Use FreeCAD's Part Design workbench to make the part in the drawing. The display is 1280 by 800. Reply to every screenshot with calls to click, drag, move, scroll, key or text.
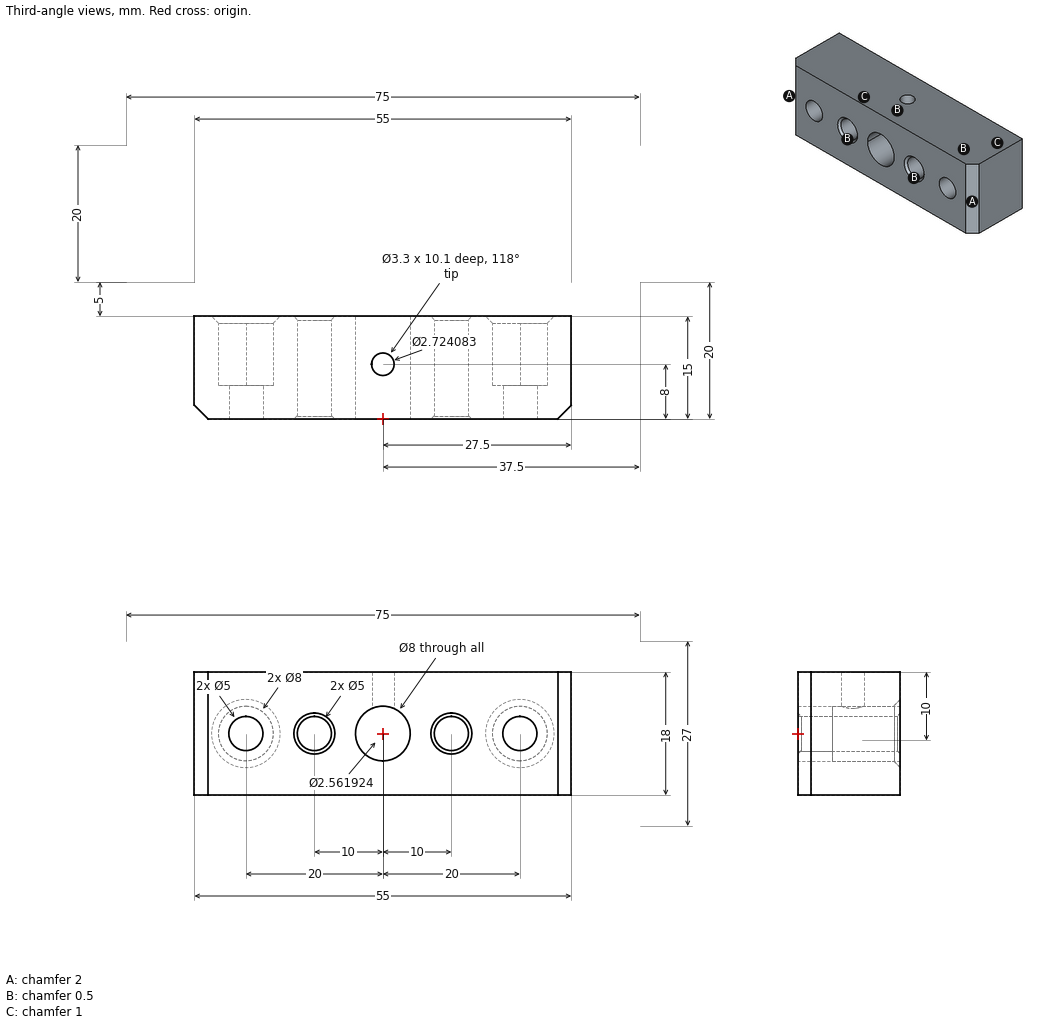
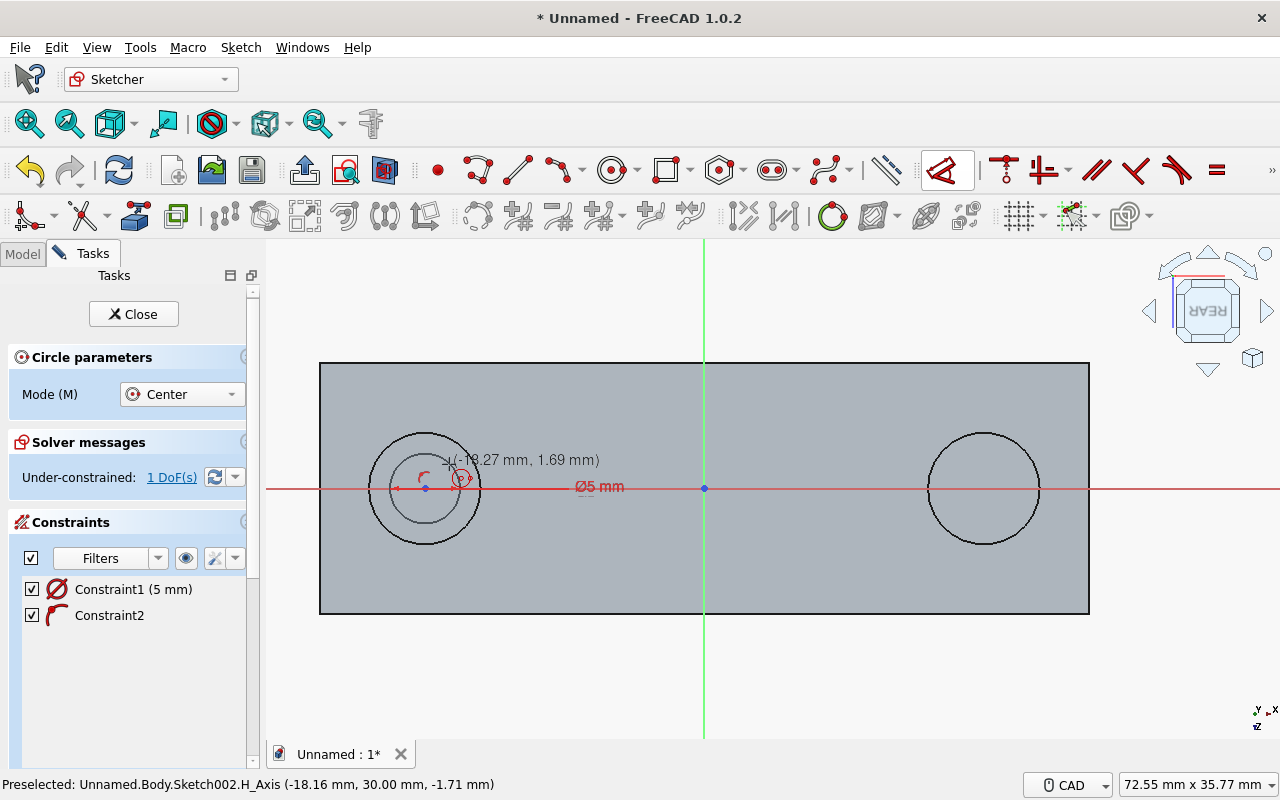
click(984, 489)
move(1009, 464)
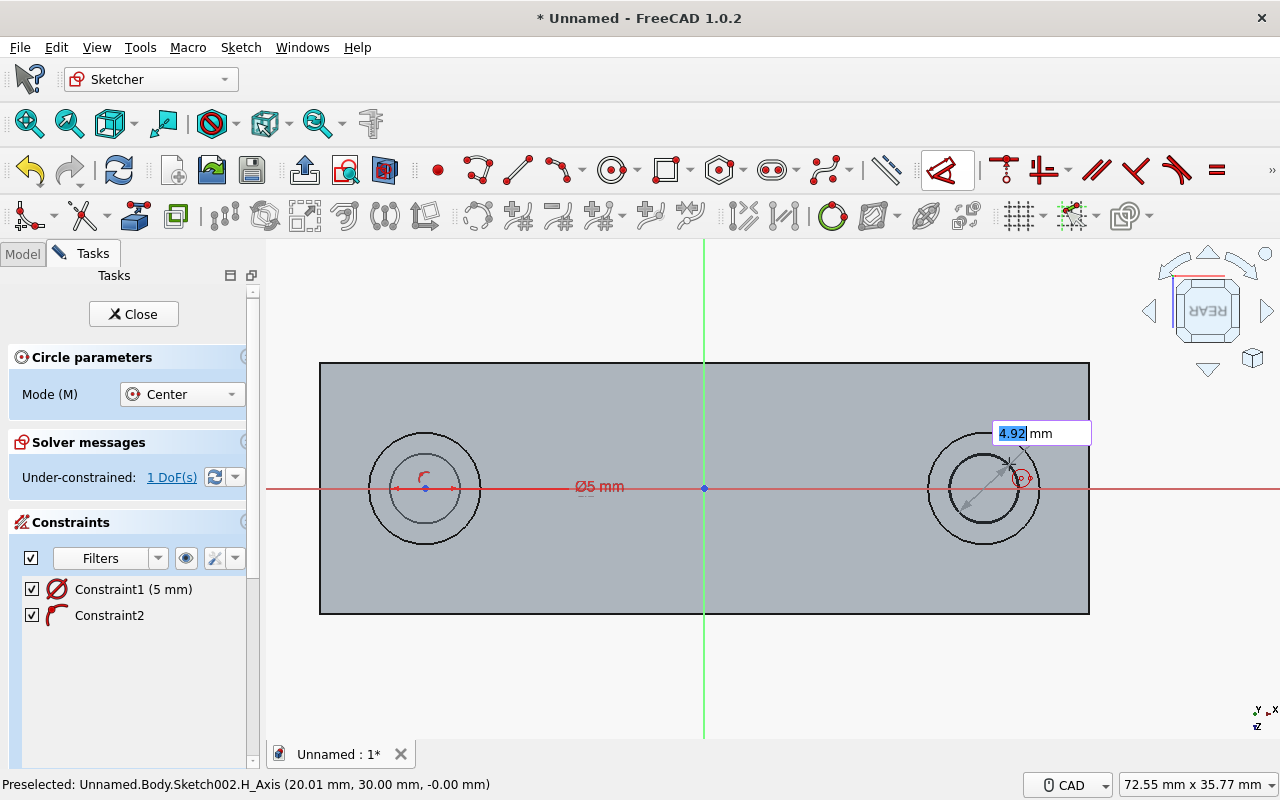
text(5)
key(Return)
key(Escape)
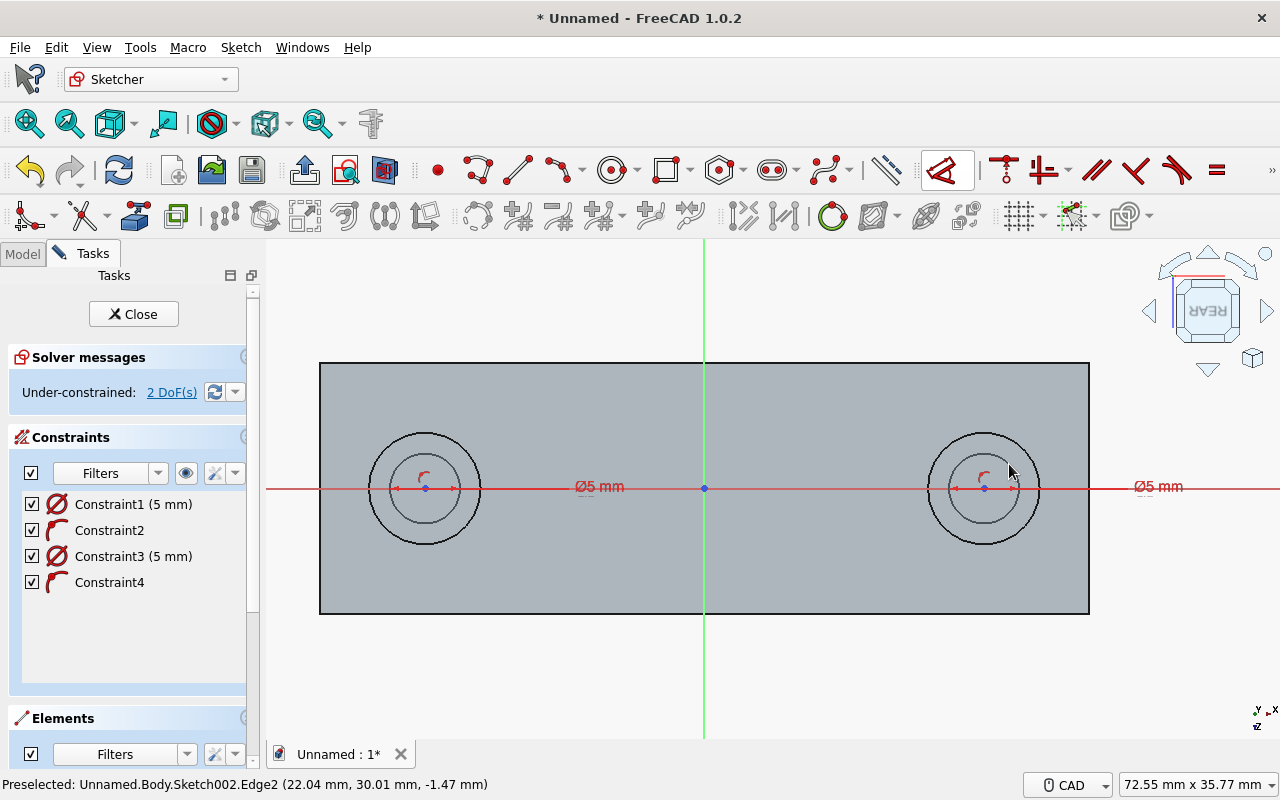
click(425, 489)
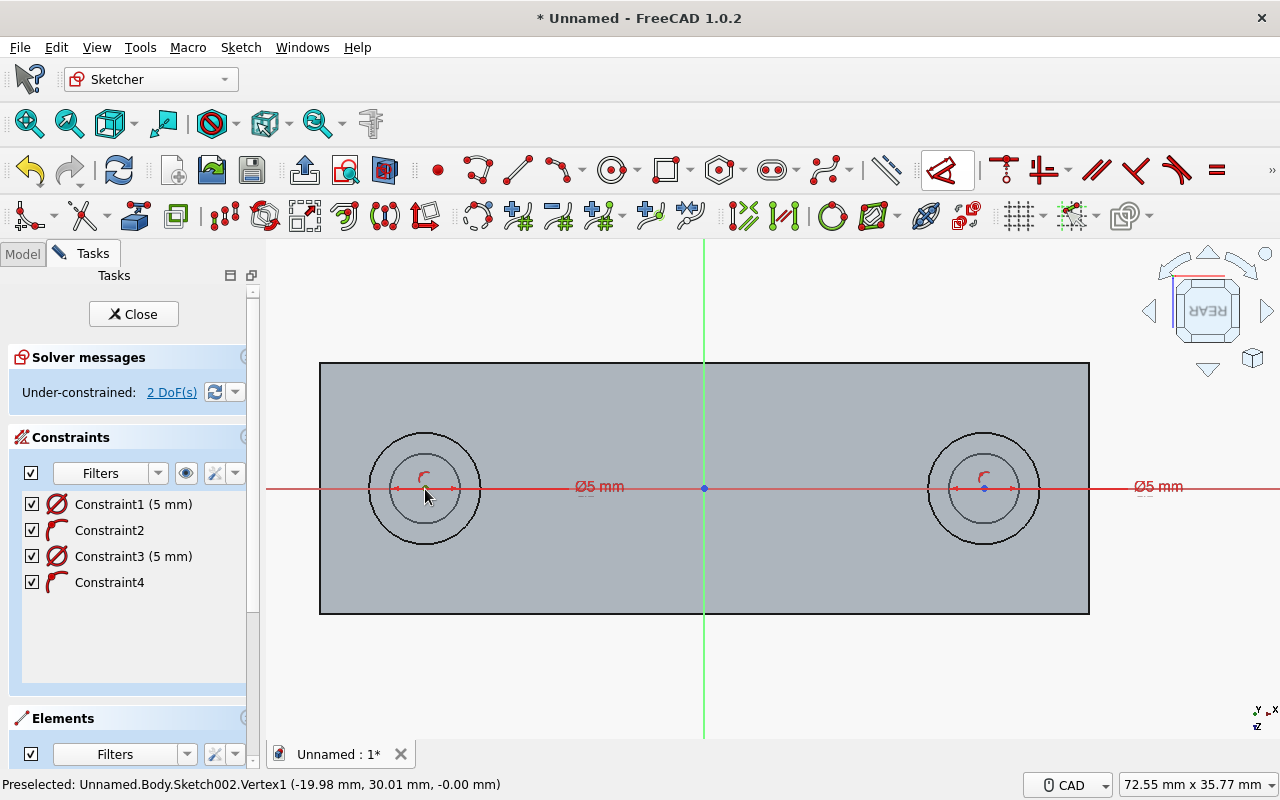
key(l)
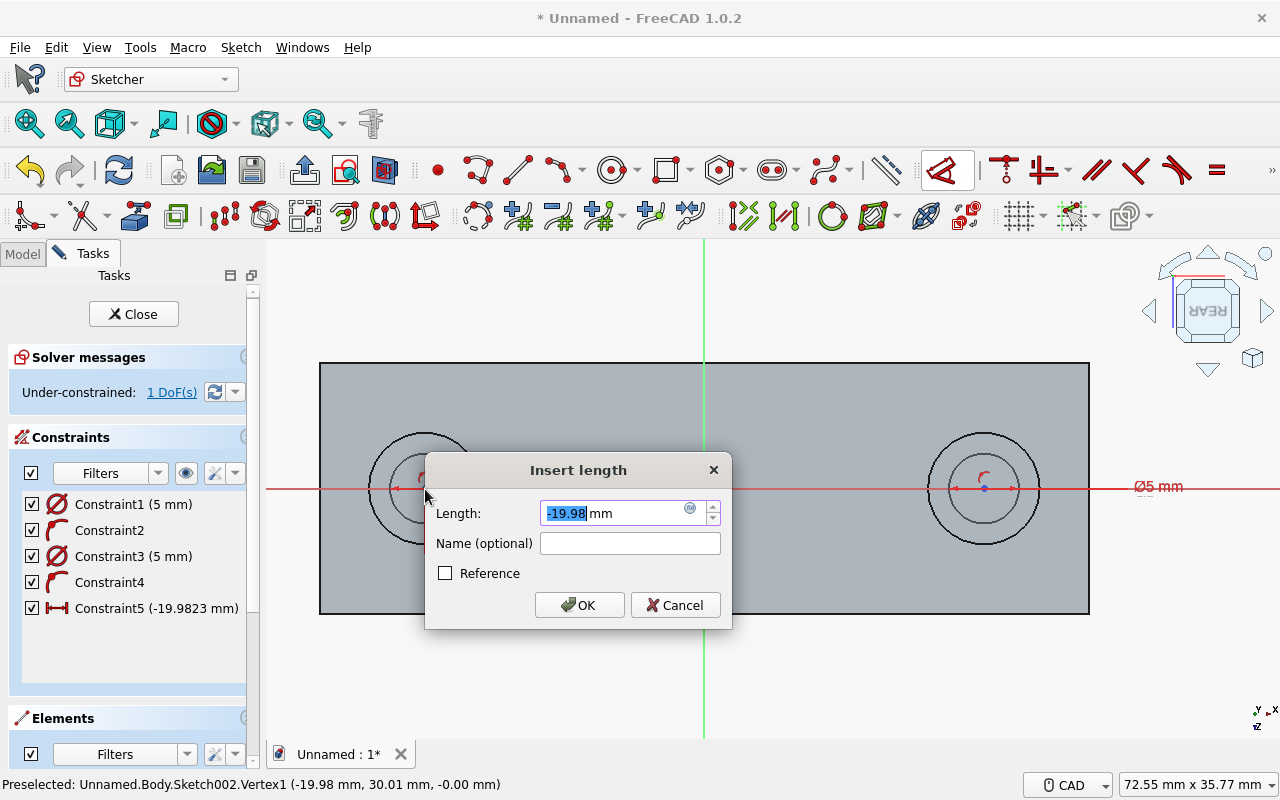
text(-20)
key(Return)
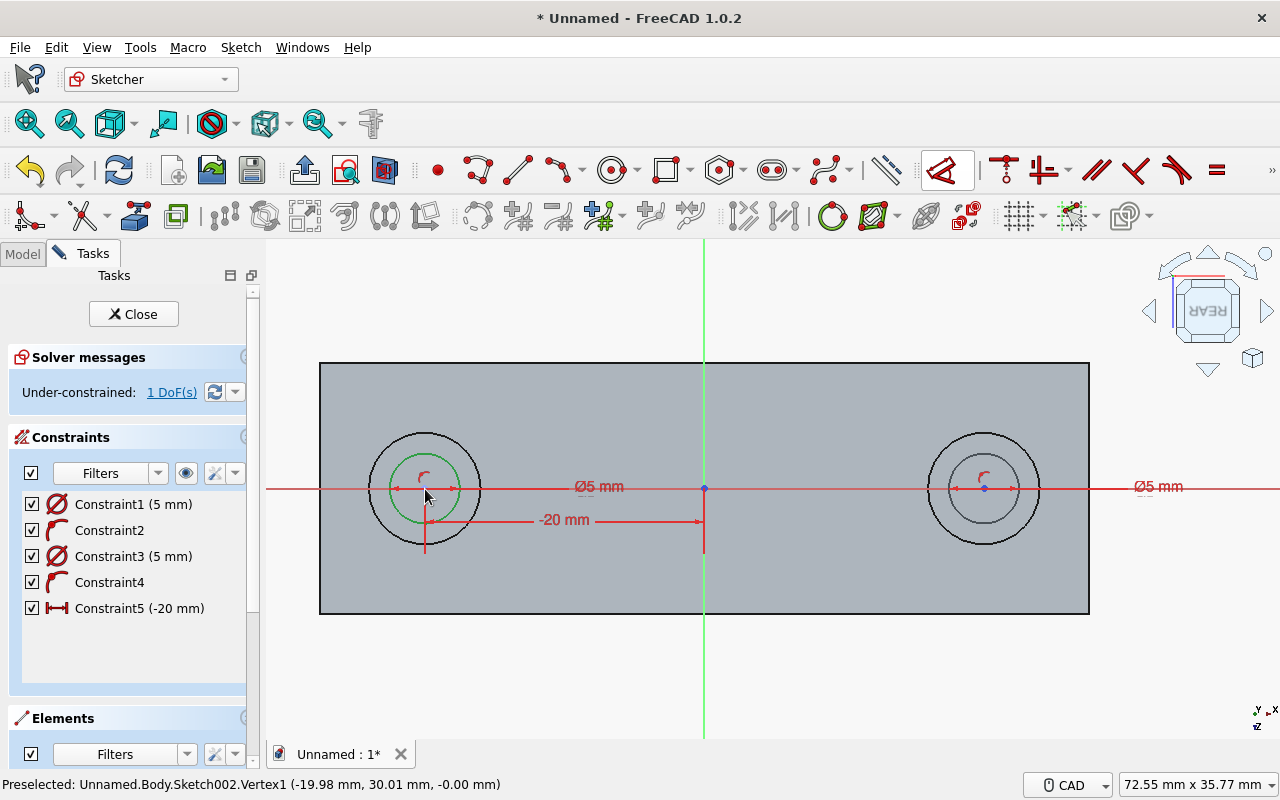
click(984, 489)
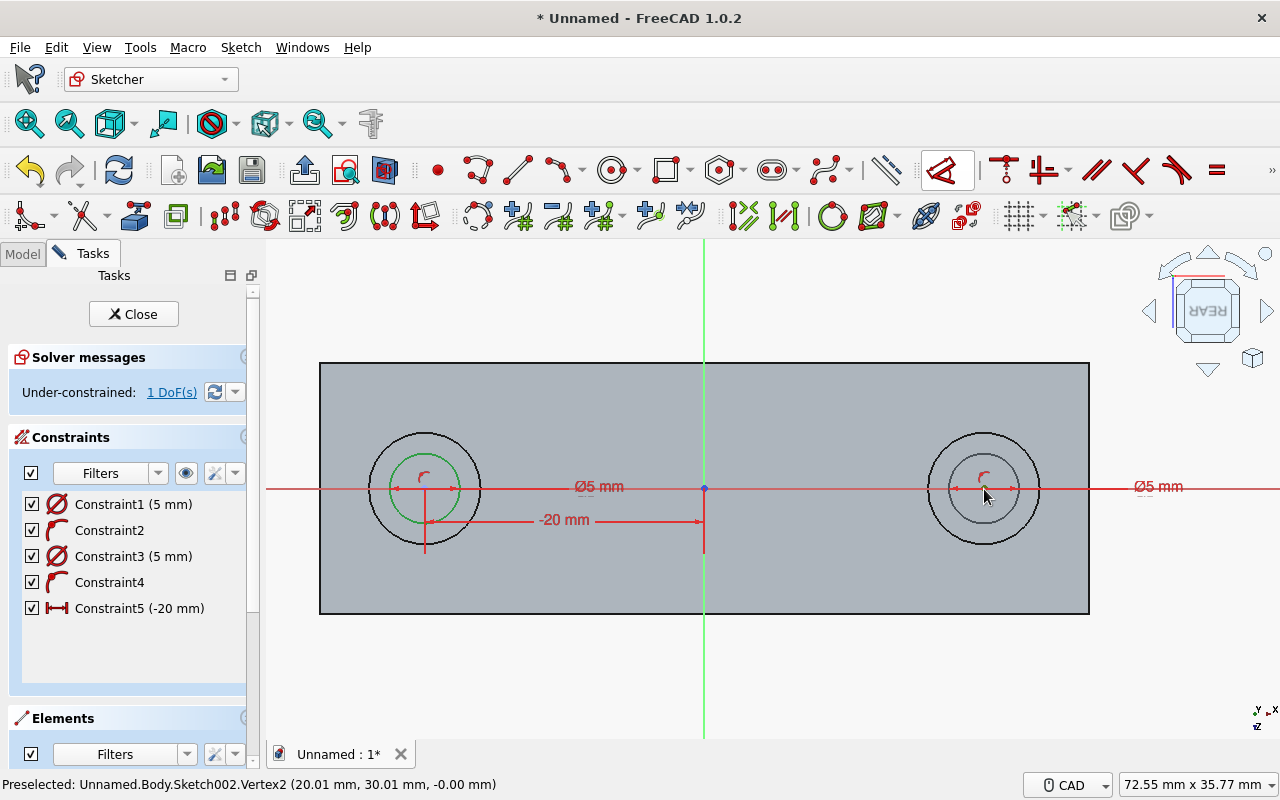
click(968, 170)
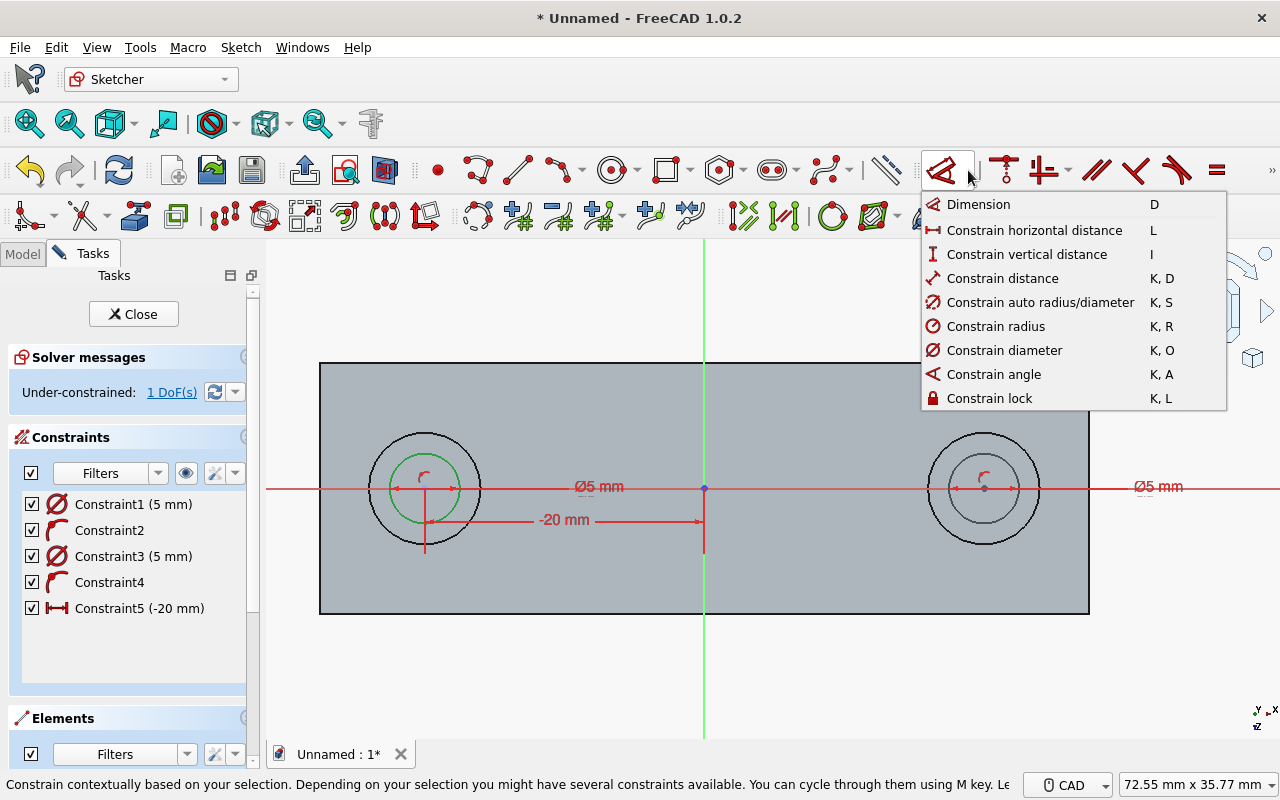
click(1074, 230)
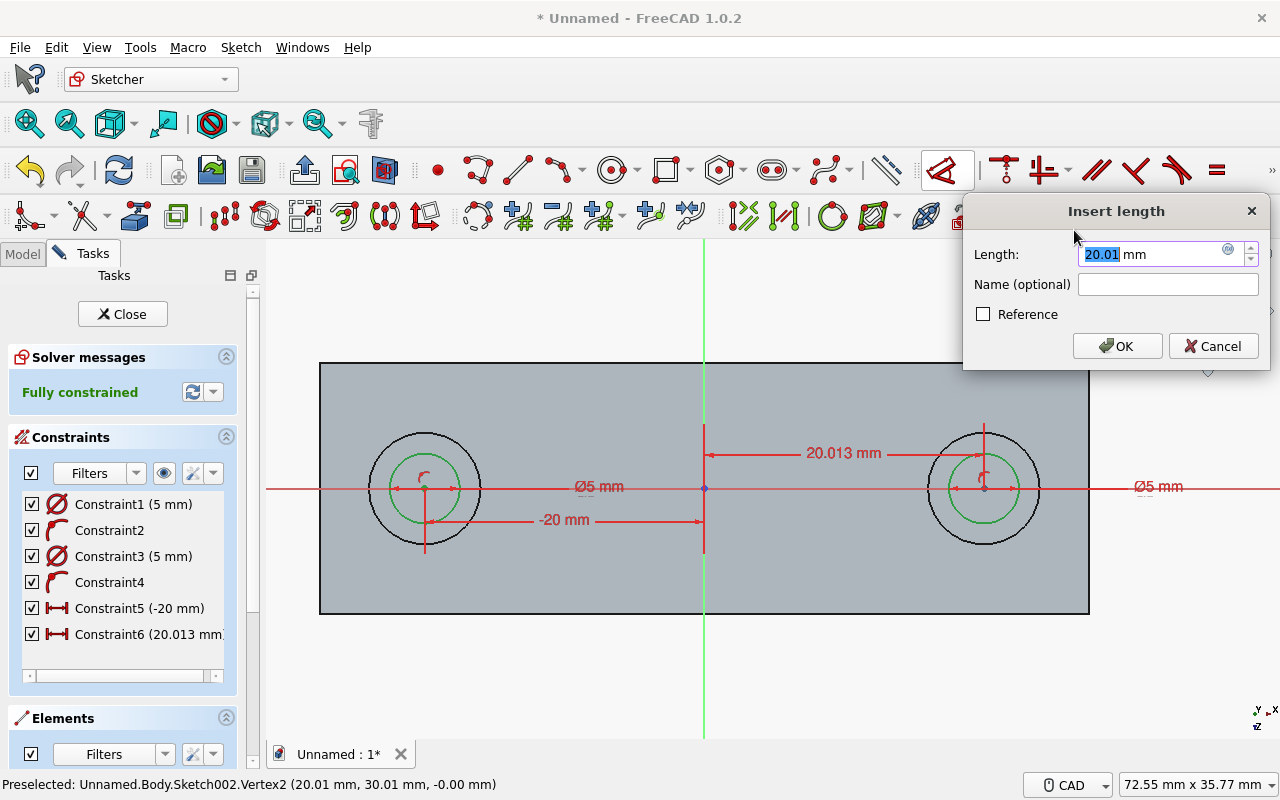
text(20)
key(Return)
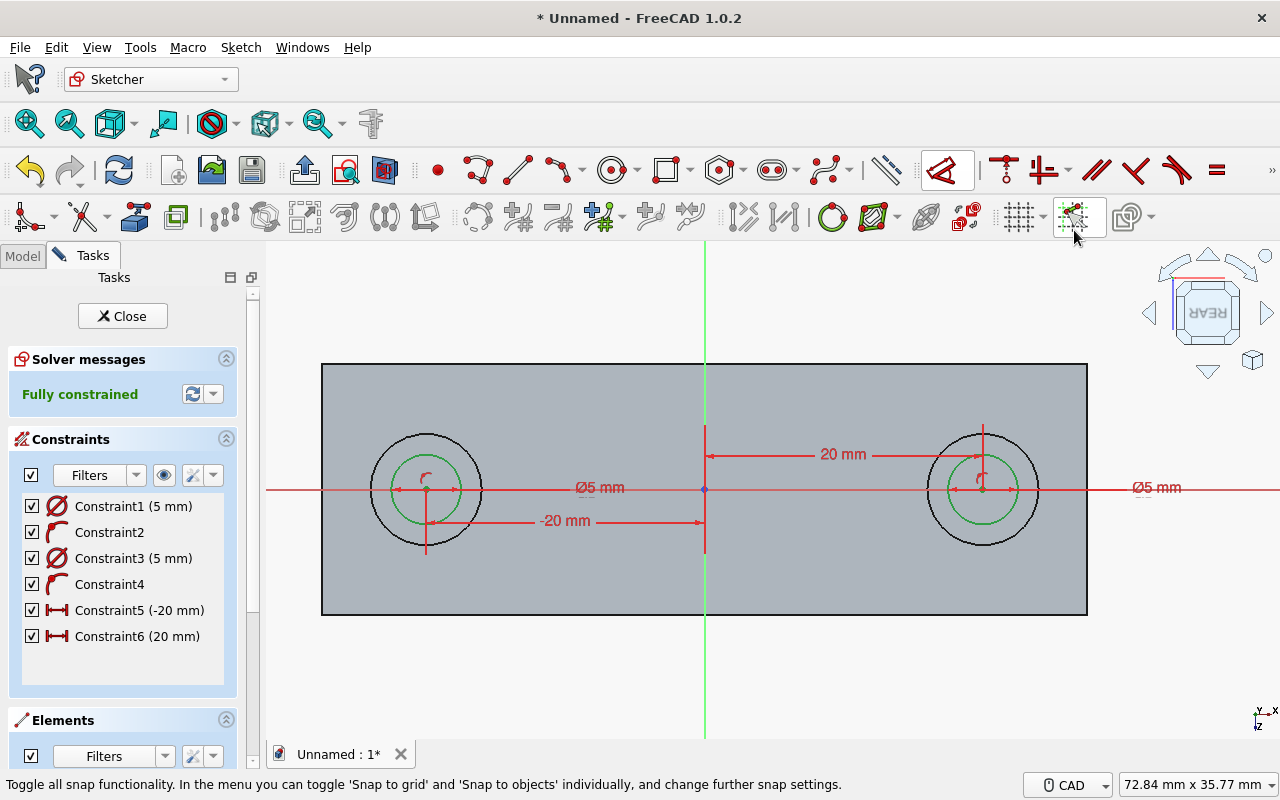
click(123, 316)